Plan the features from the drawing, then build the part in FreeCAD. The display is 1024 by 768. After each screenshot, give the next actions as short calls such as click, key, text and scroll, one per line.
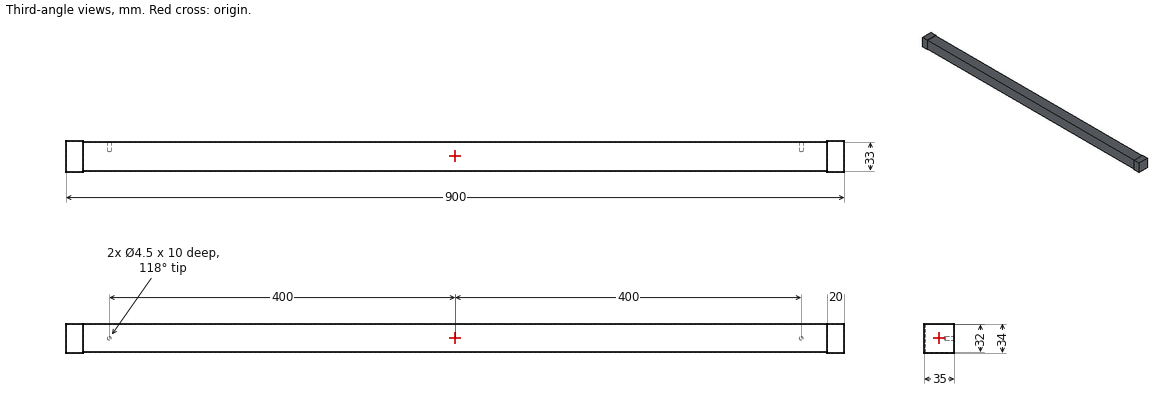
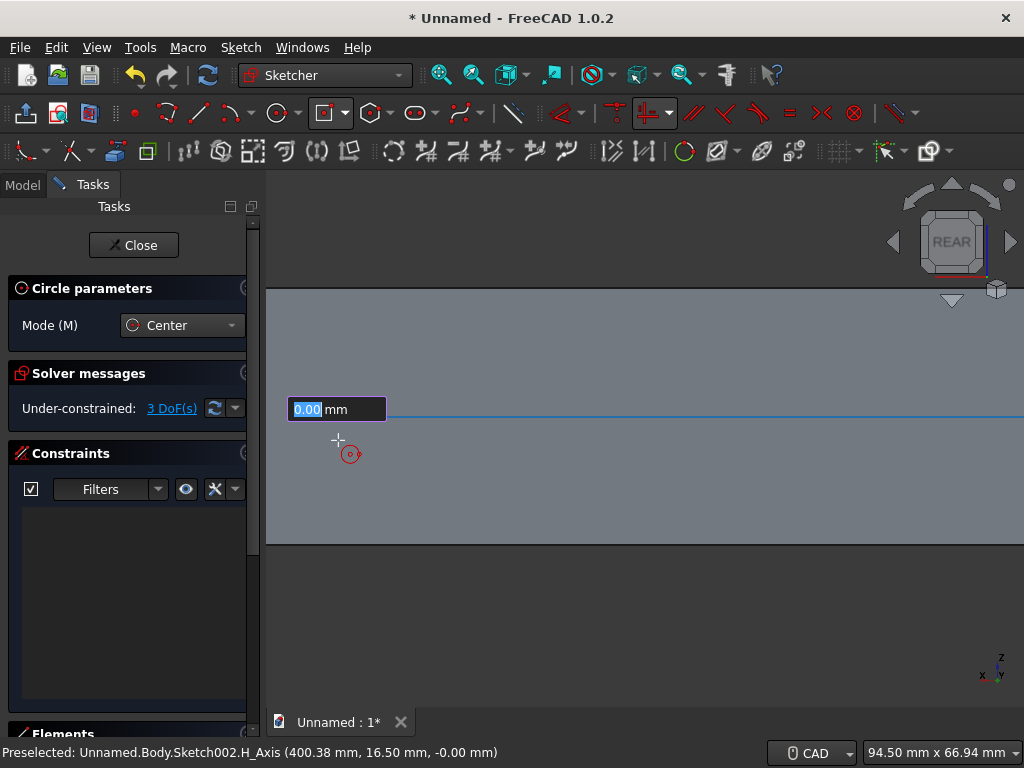
click(334, 434)
key(Escape)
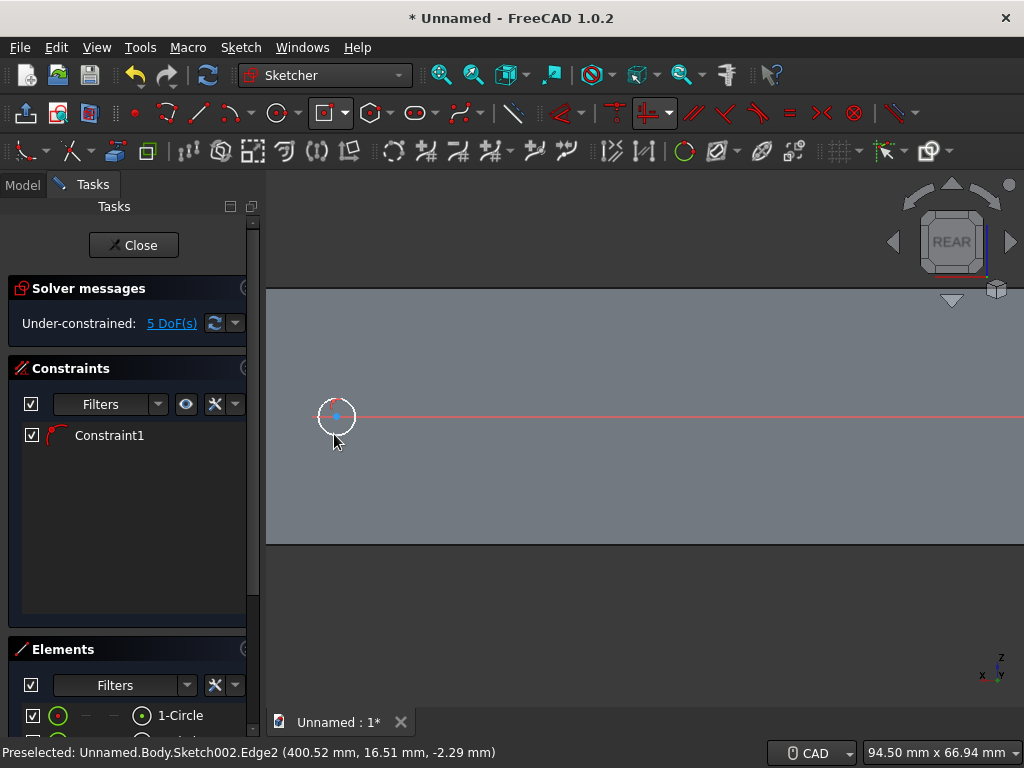
scroll(384, 440, down, 14)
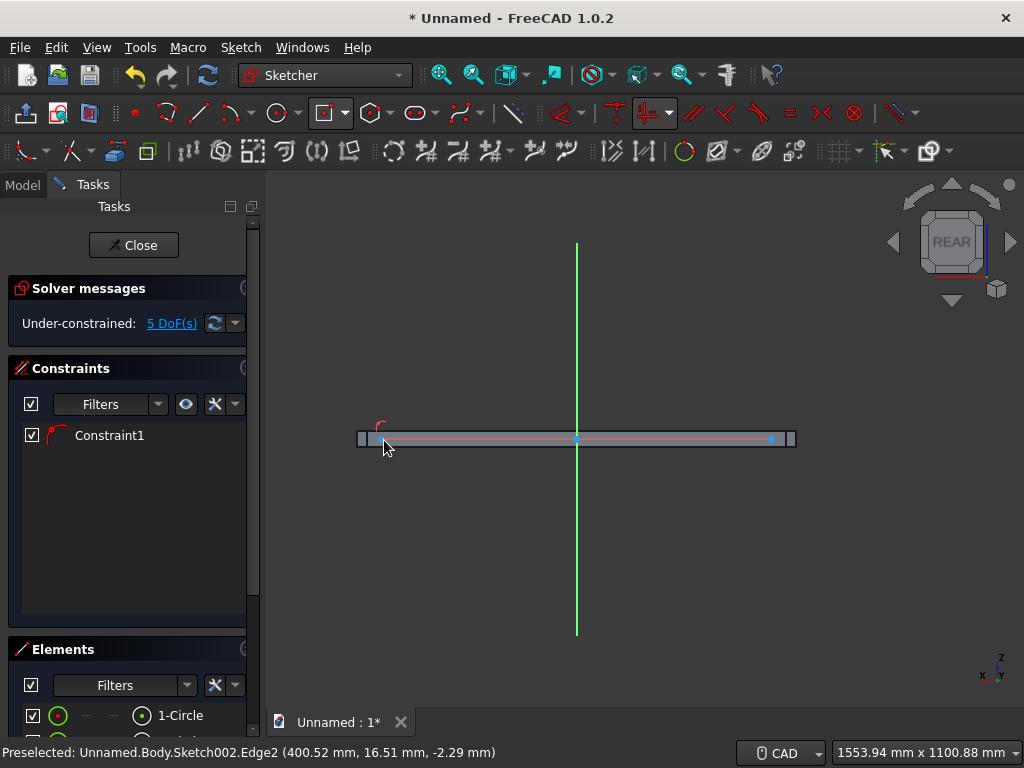
scroll(772, 439, up, 14)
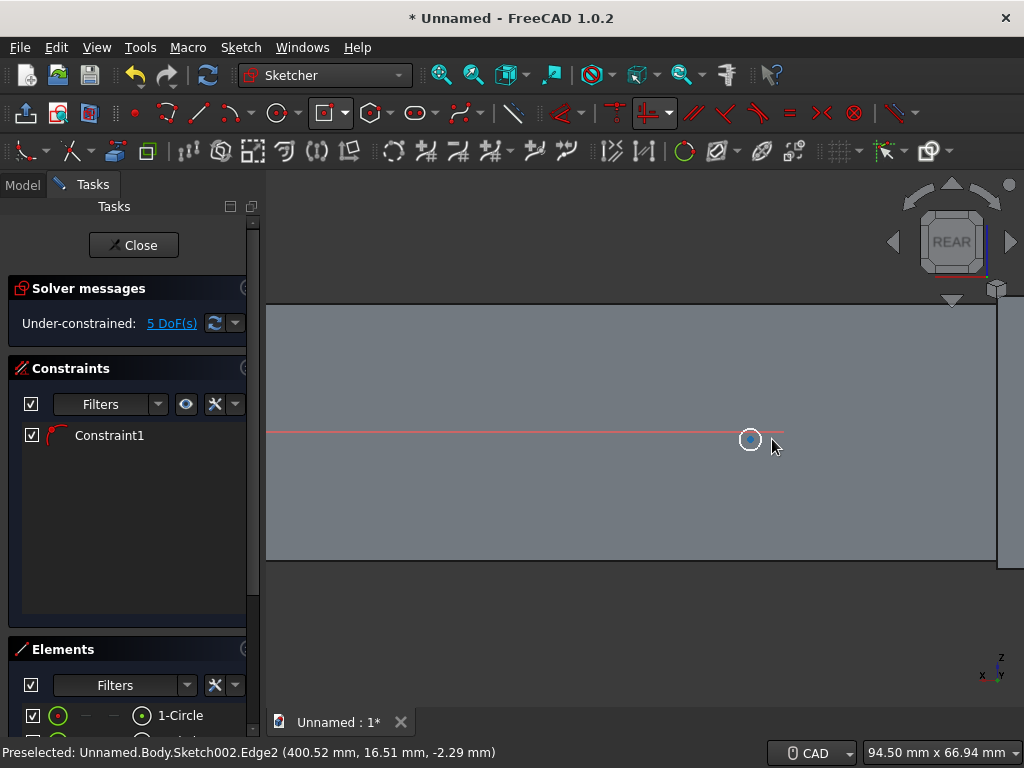
click(758, 432)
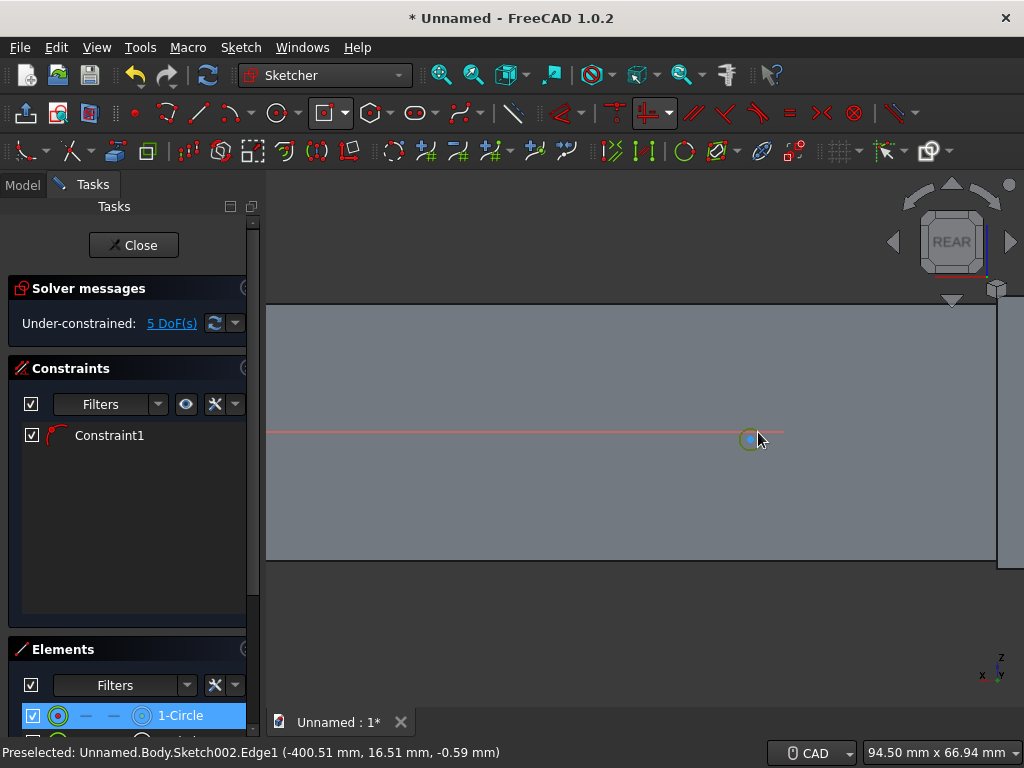
scroll(773, 439, down, 14)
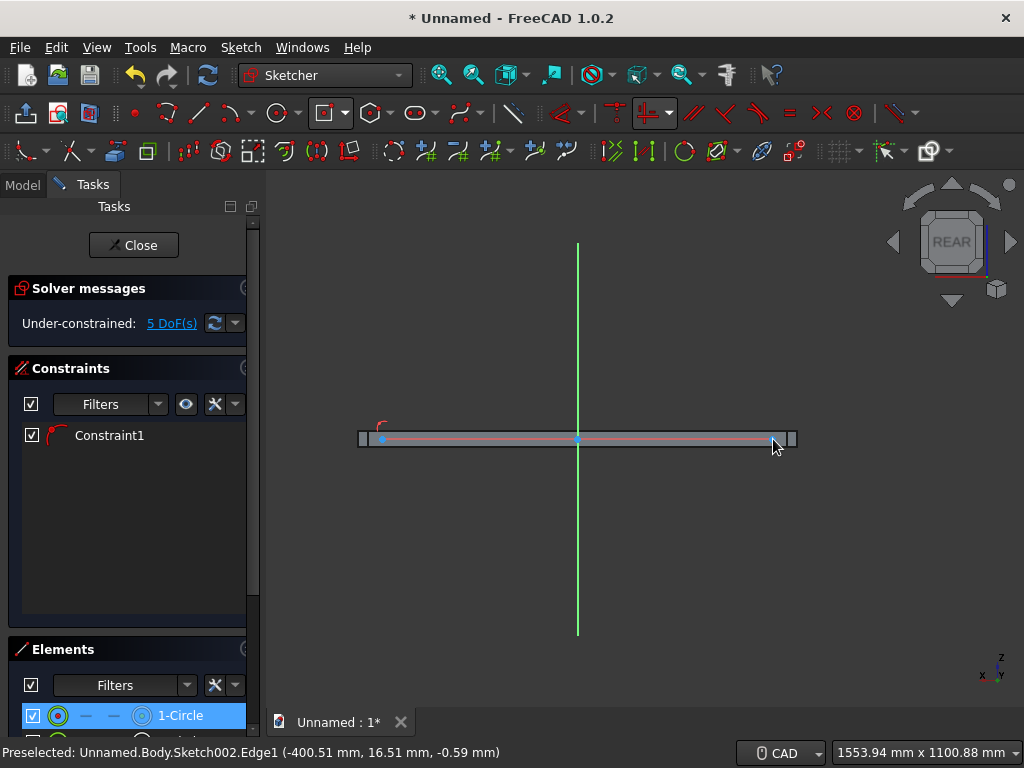
scroll(383, 438, up, 14)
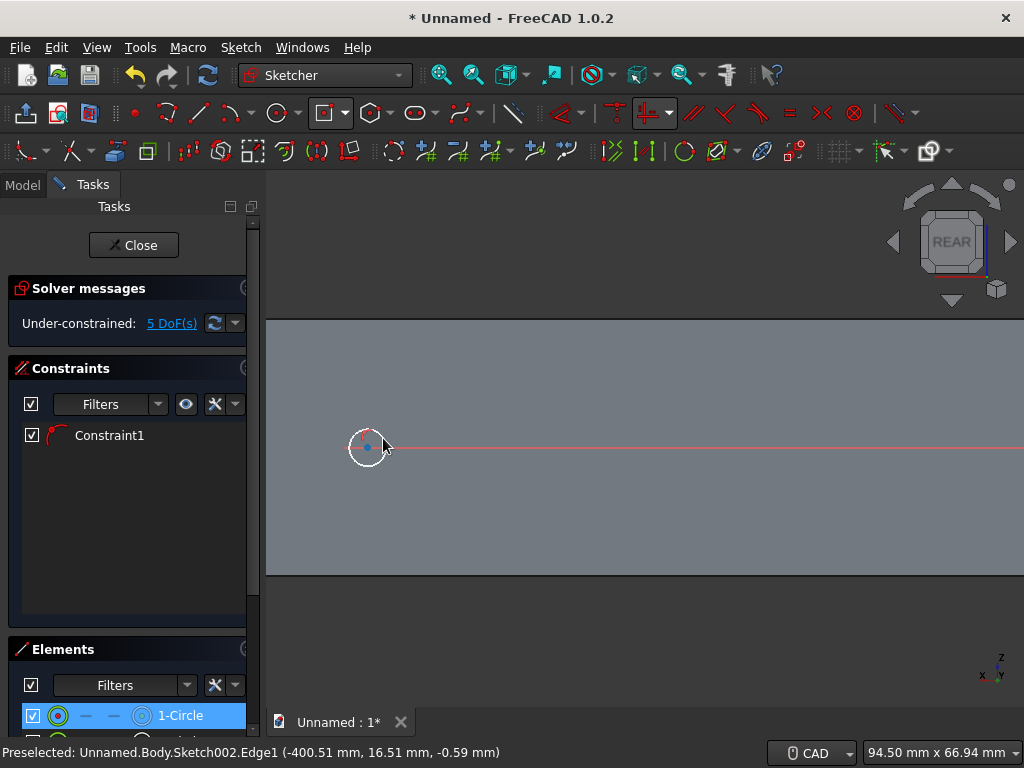
click(381, 435)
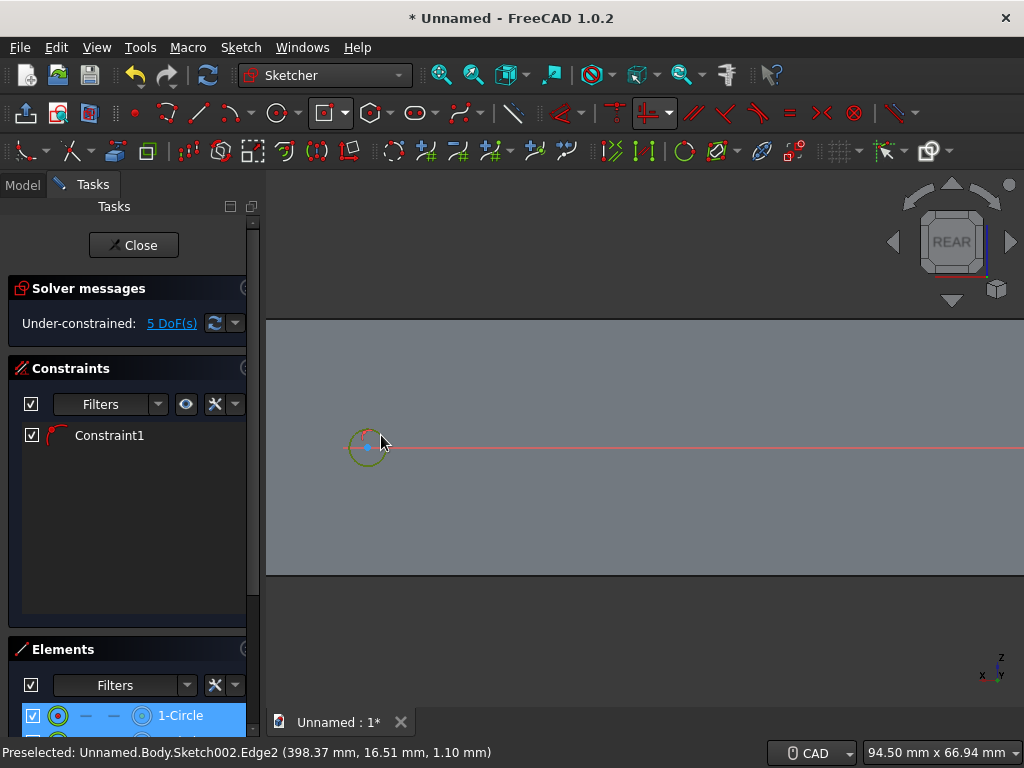
click(790, 114)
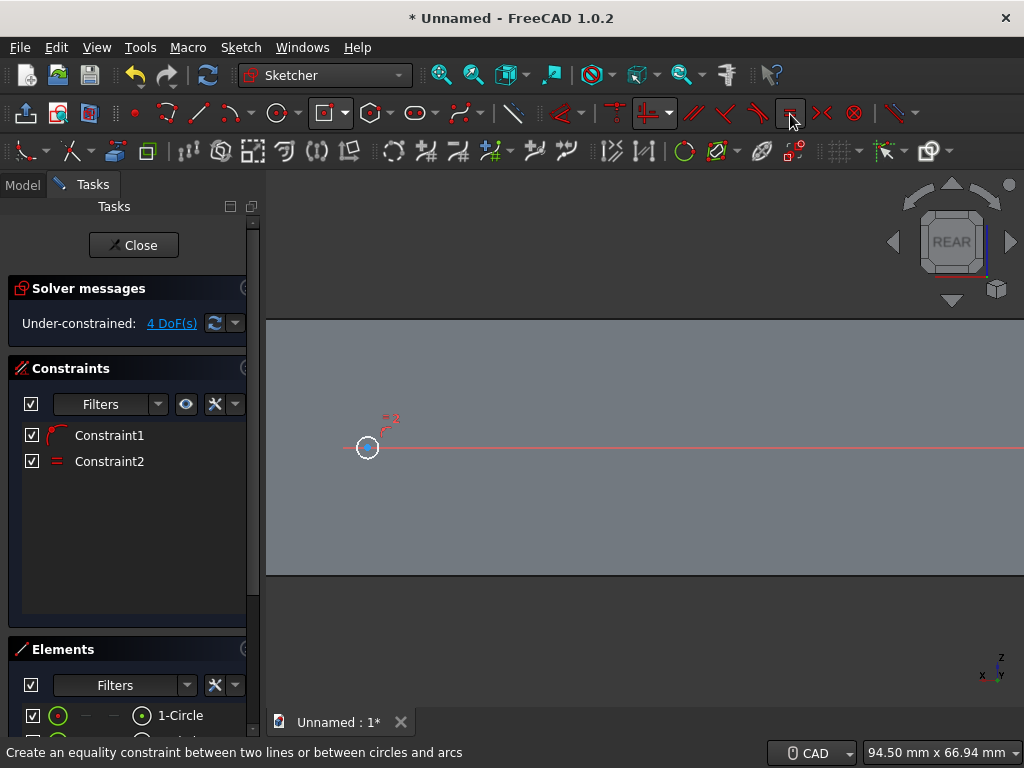
scroll(382, 438, down, 14)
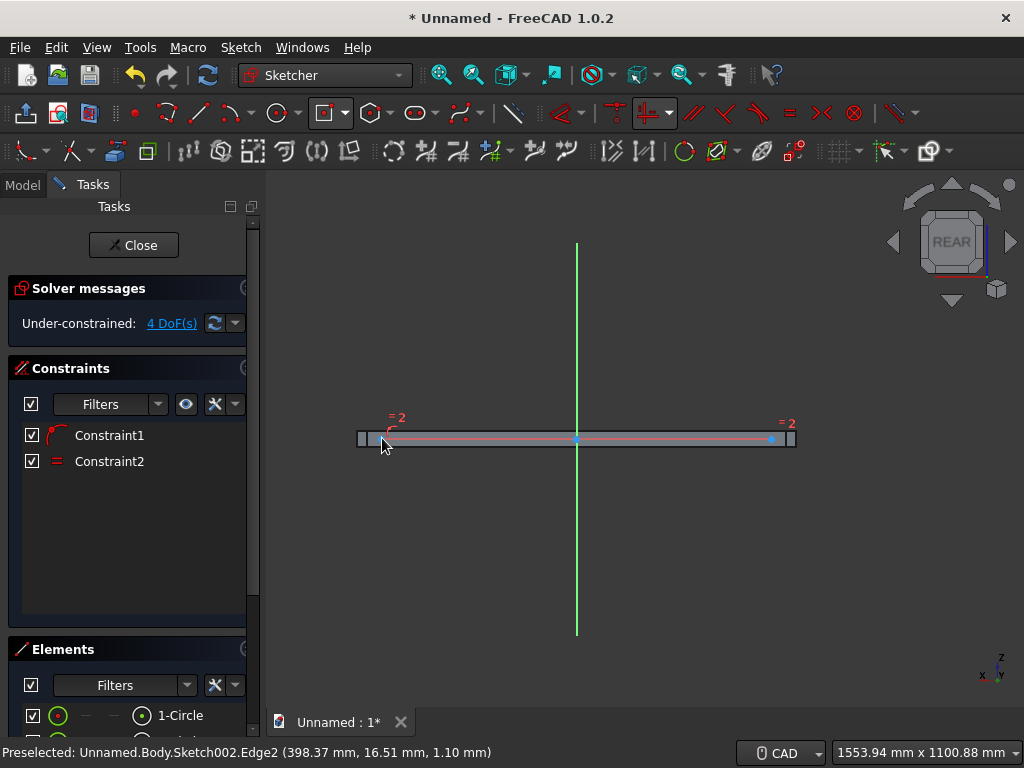
click(771, 440)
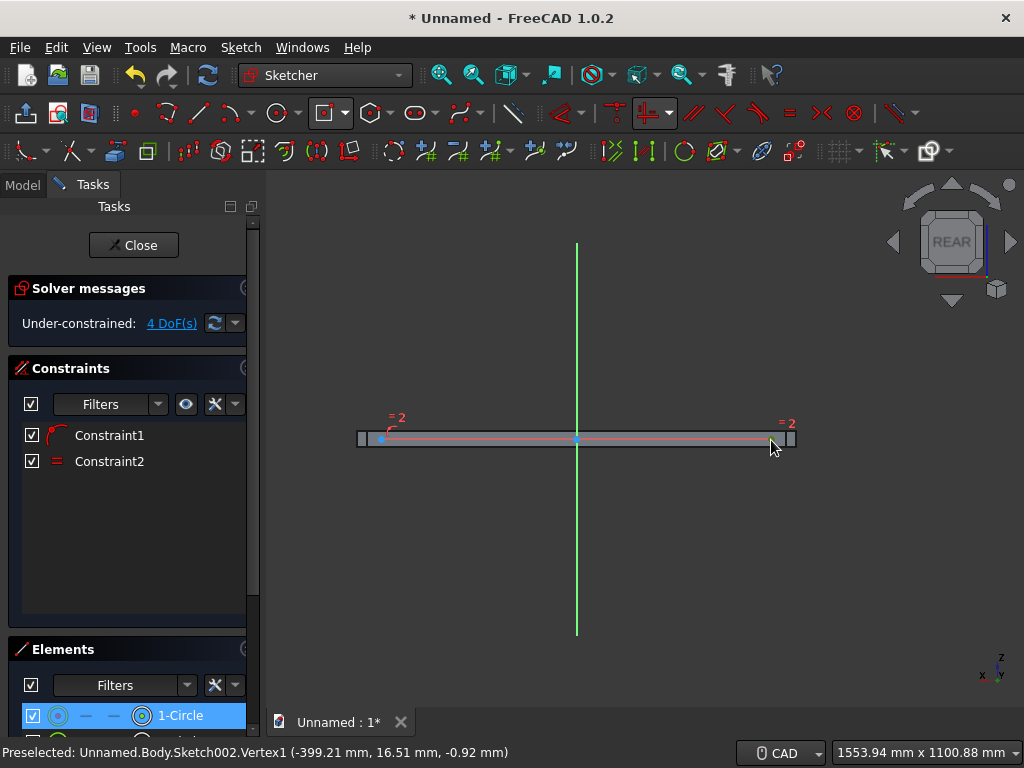
click(415, 439)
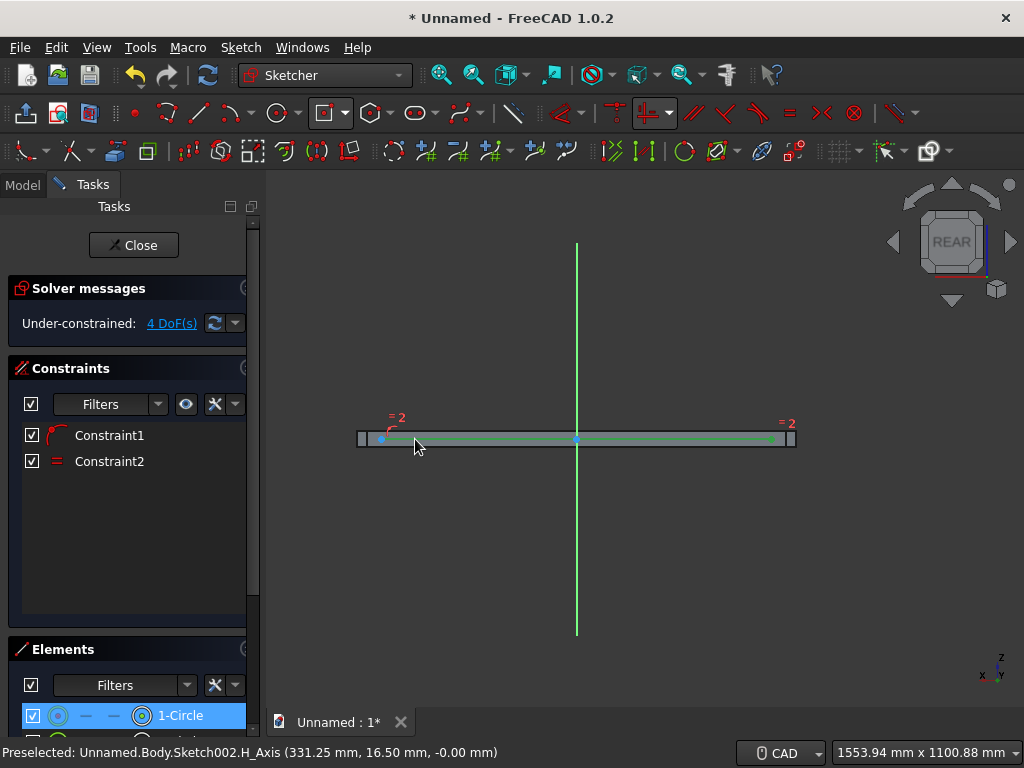
key(c)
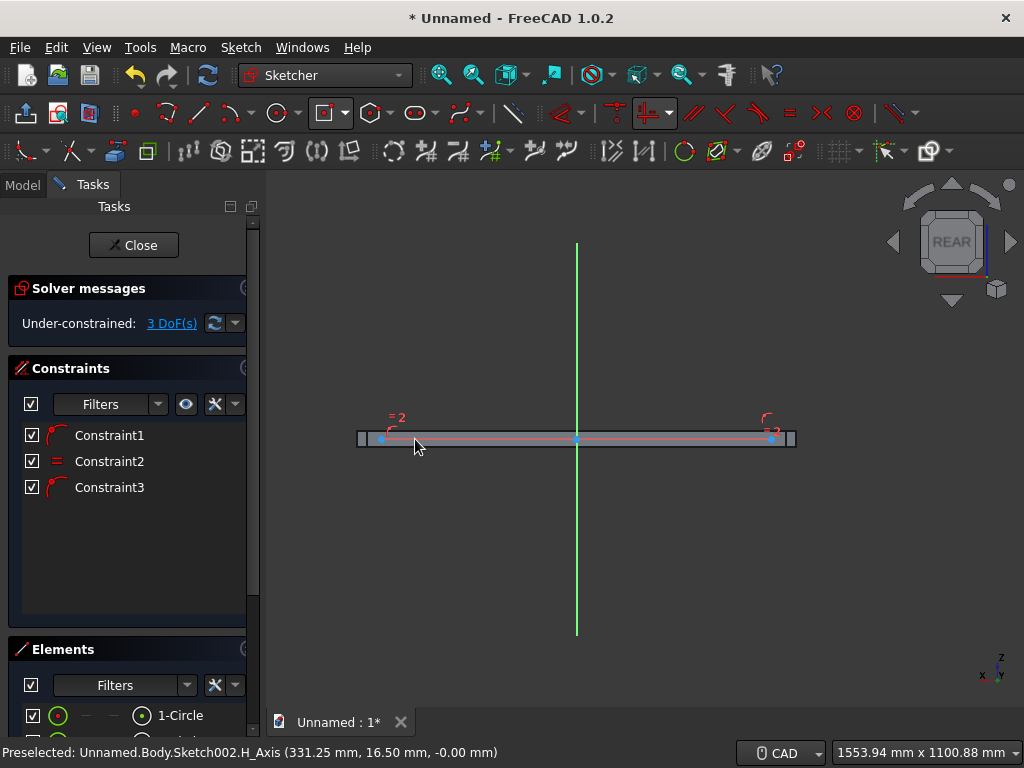
scroll(772, 440, up, 15)